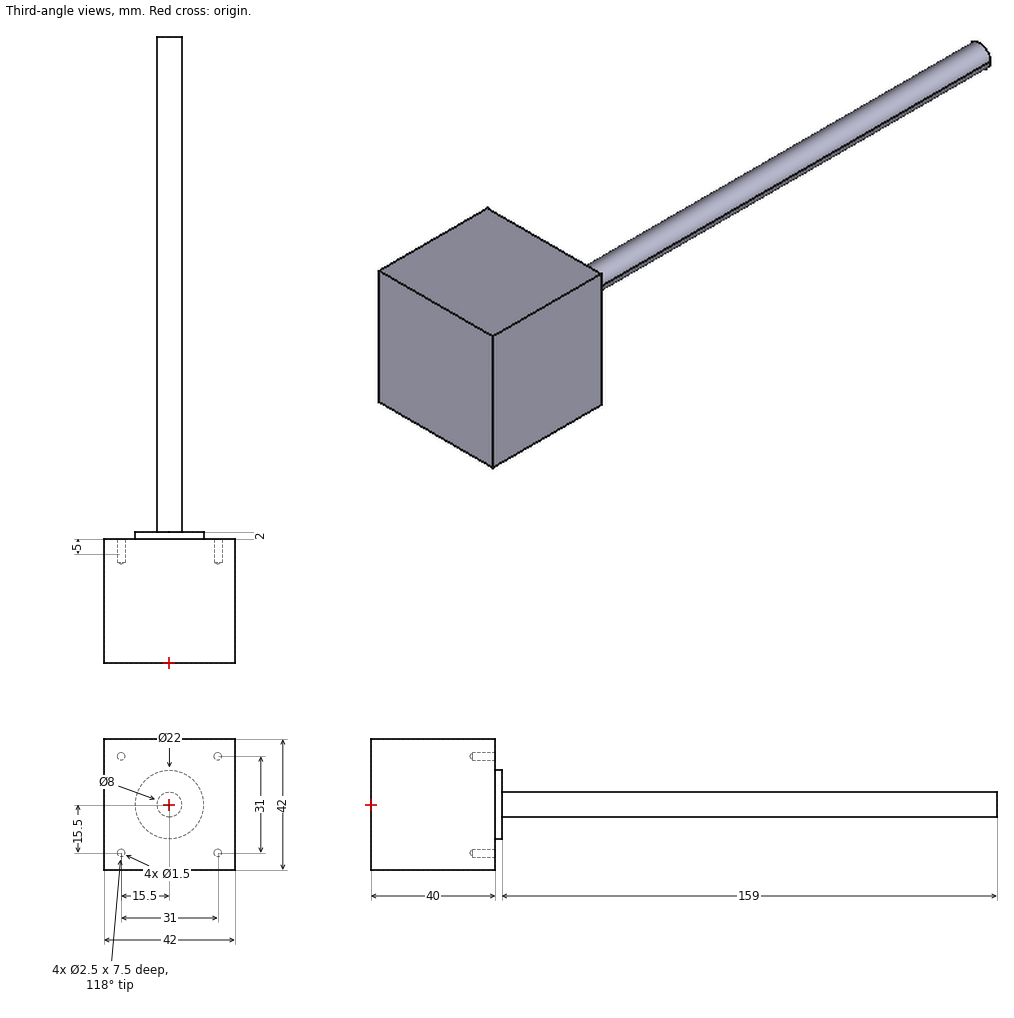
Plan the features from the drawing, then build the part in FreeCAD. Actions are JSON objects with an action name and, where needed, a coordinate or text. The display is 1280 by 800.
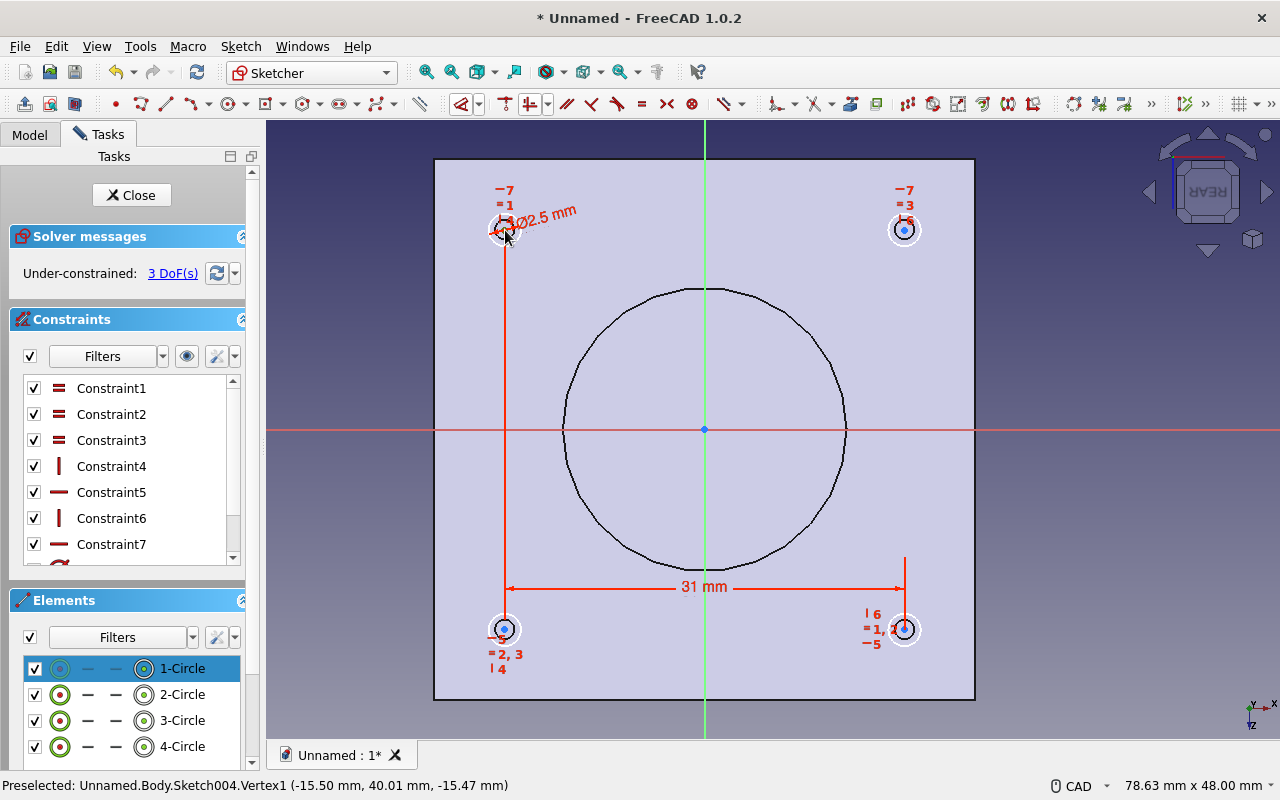
{"action": "left_click", "coordinate": [905, 630]}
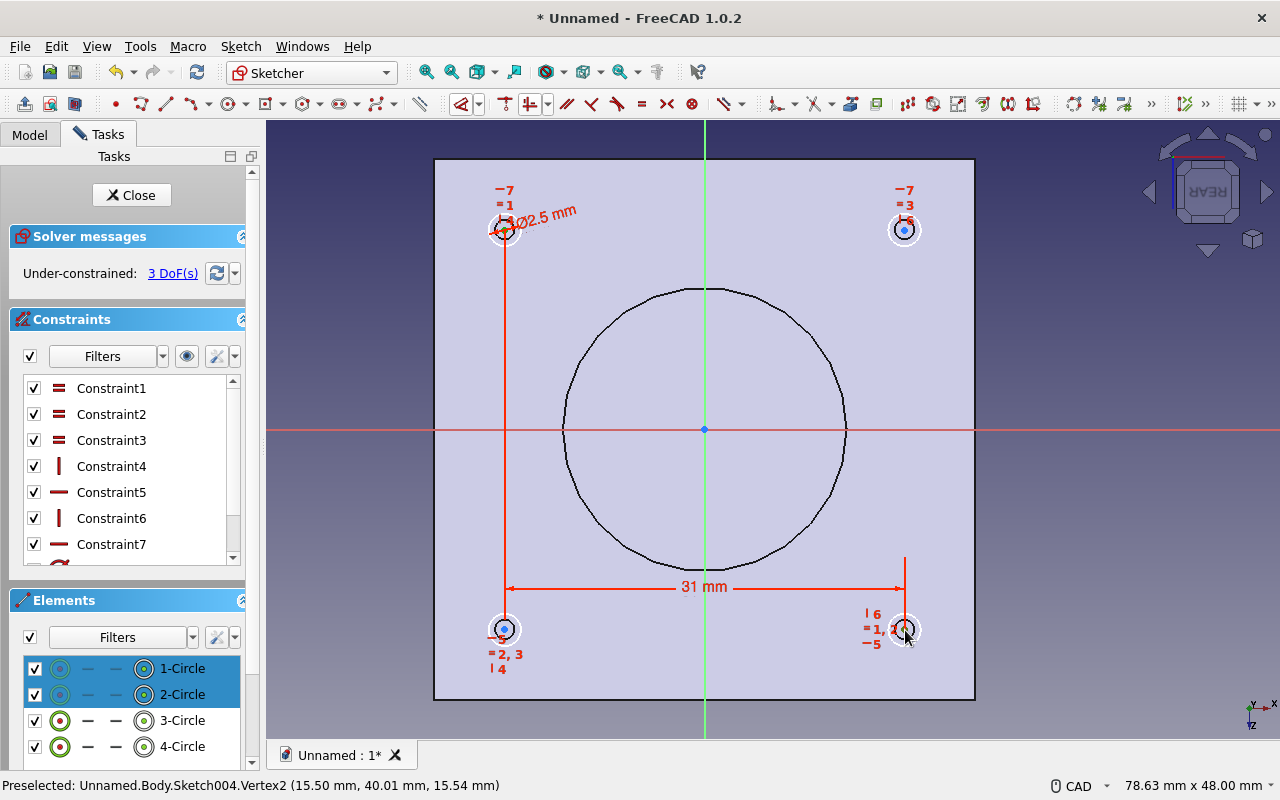
{"action": "key", "text": "i"}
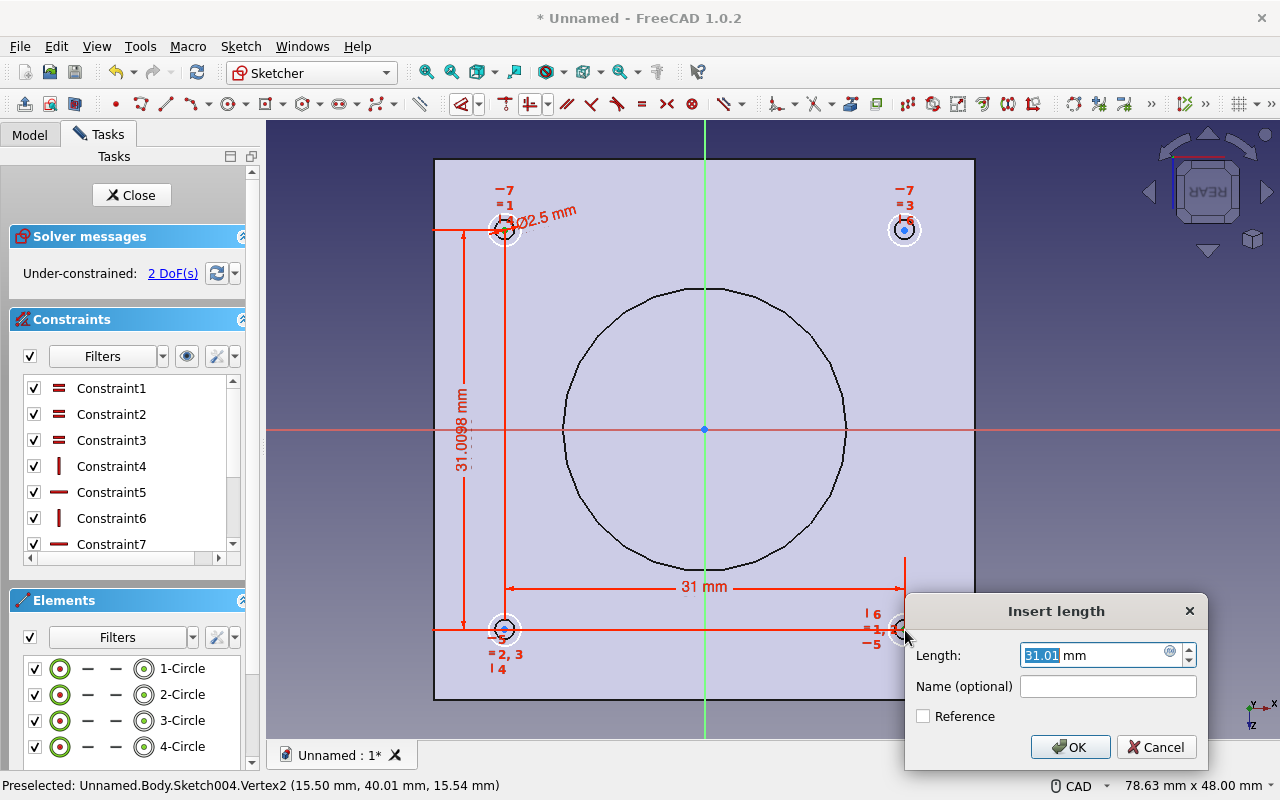
{"action": "type", "text": "31"}
{"action": "key", "text": "Return"}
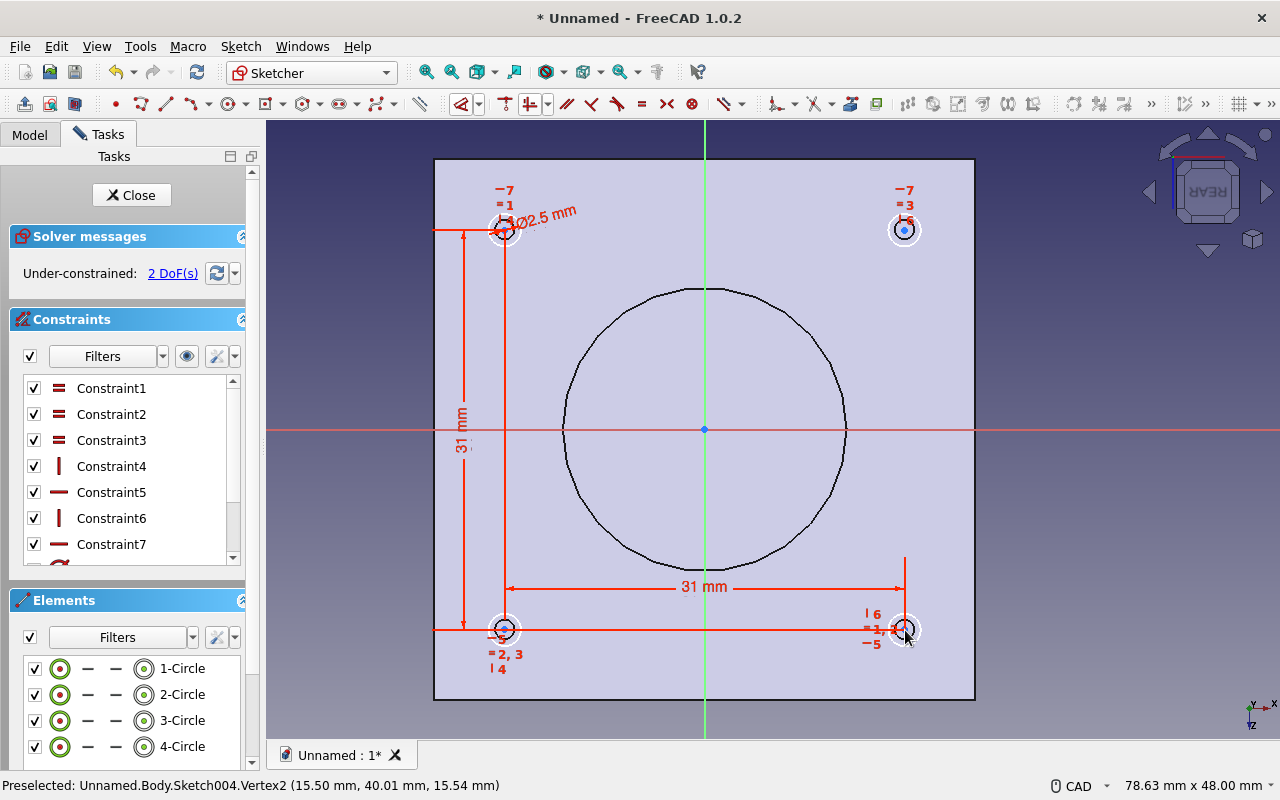
{"action": "left_click", "coordinate": [505, 230]}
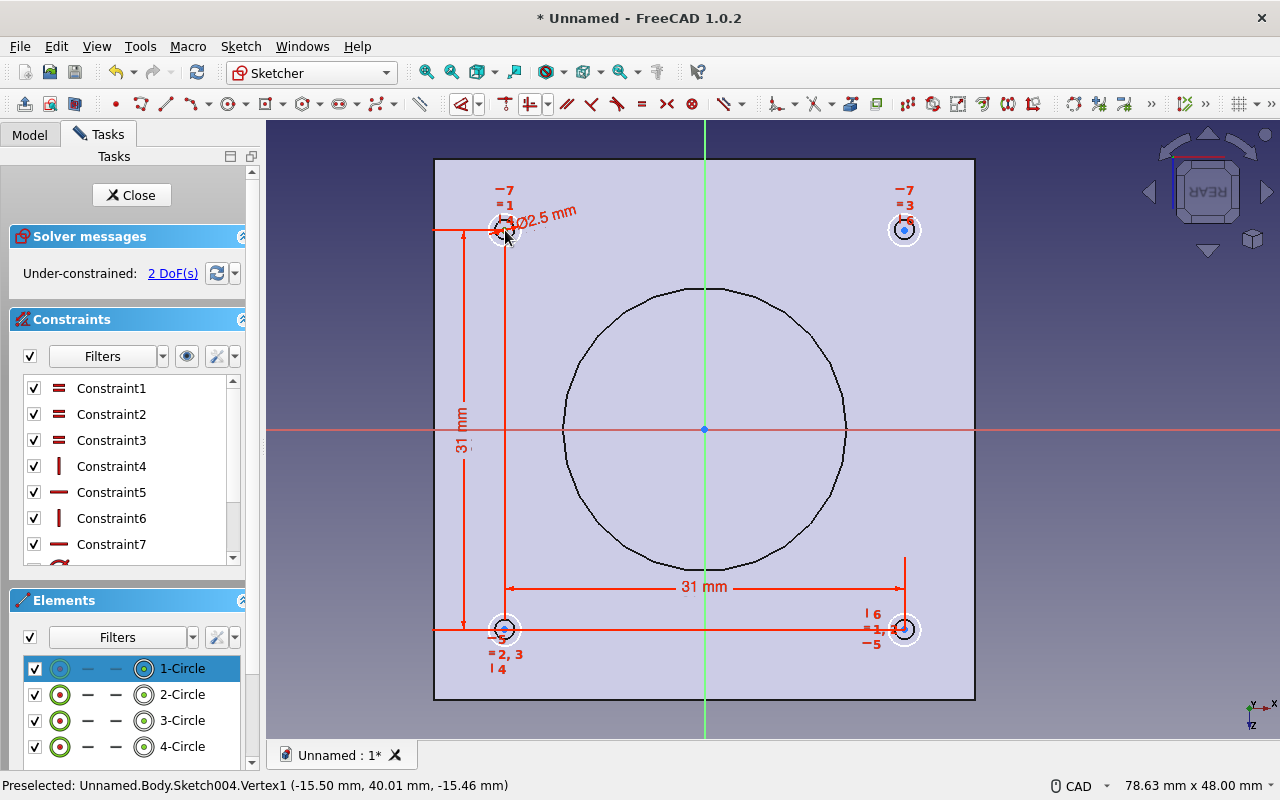
{"action": "key", "text": "l"}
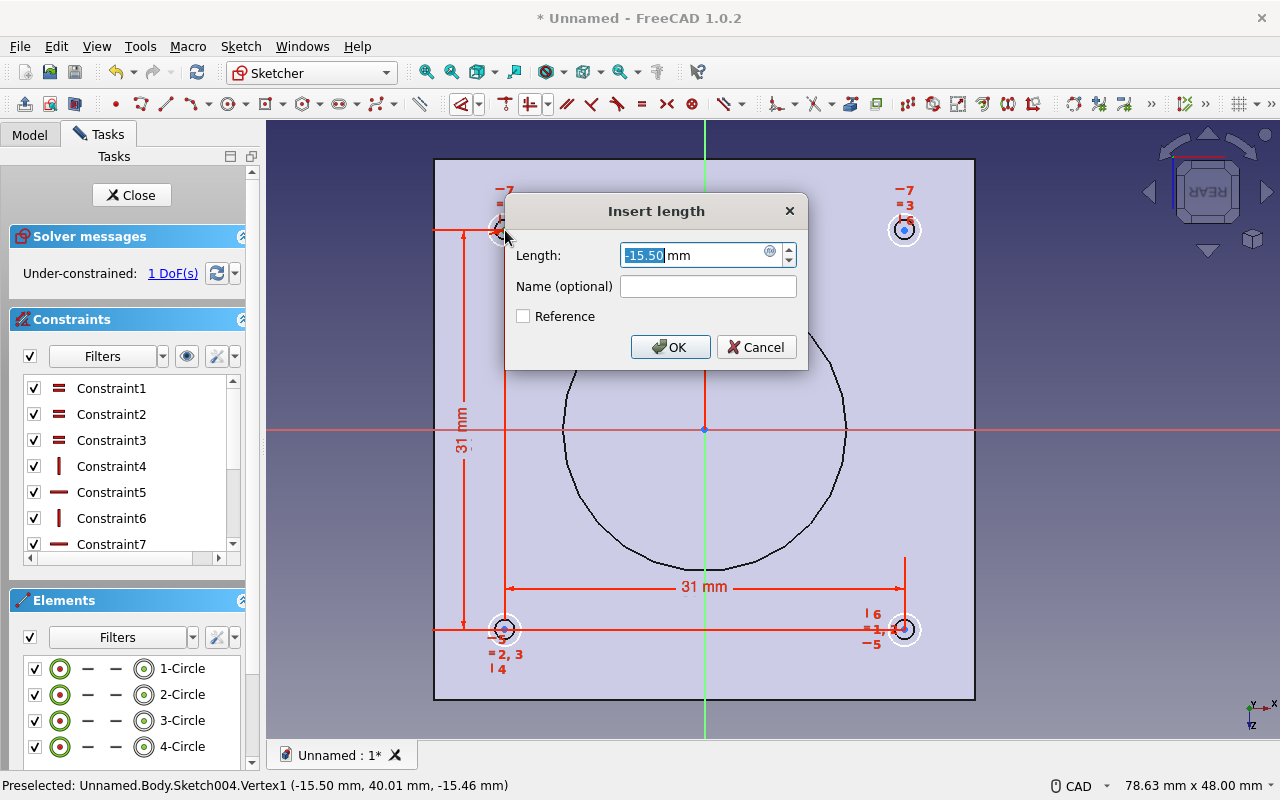
{"action": "type", "text": "-15.5"}
{"action": "key", "text": "Return"}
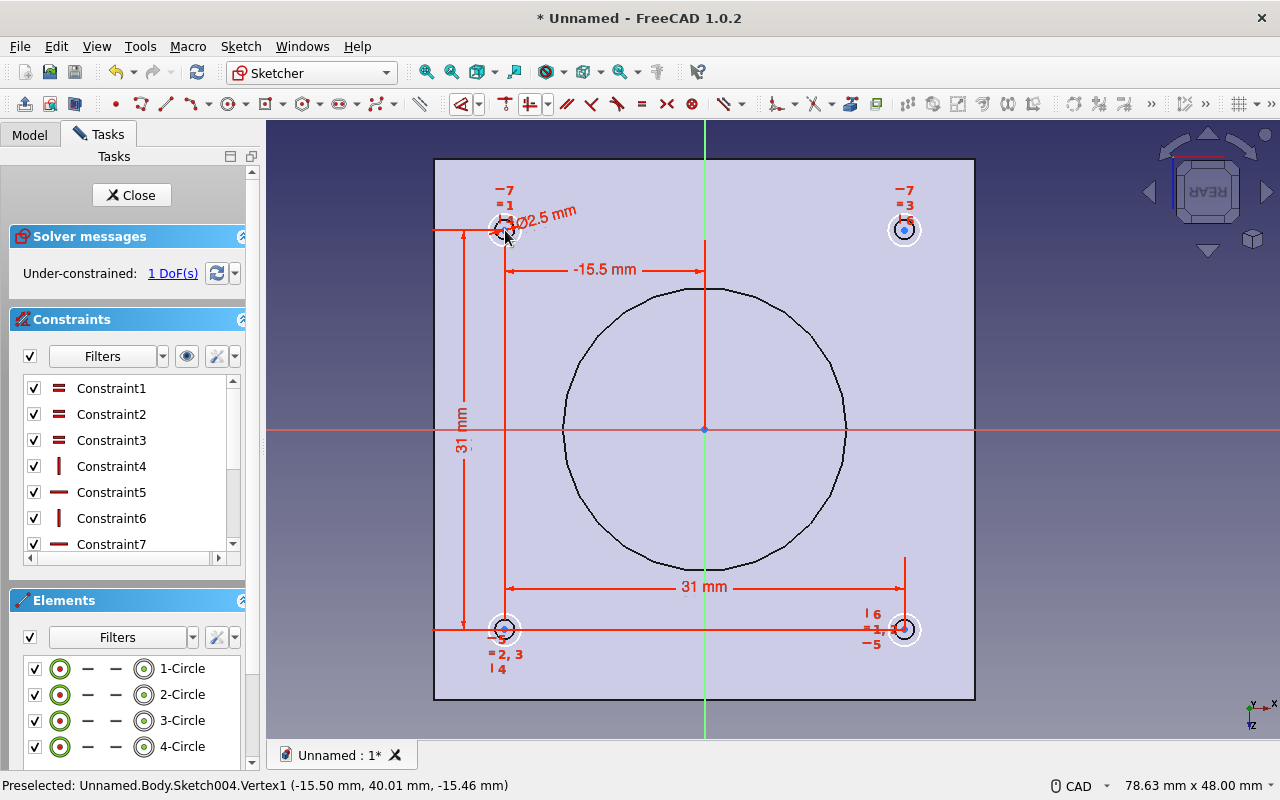
{"action": "left_click", "coordinate": [505, 230]}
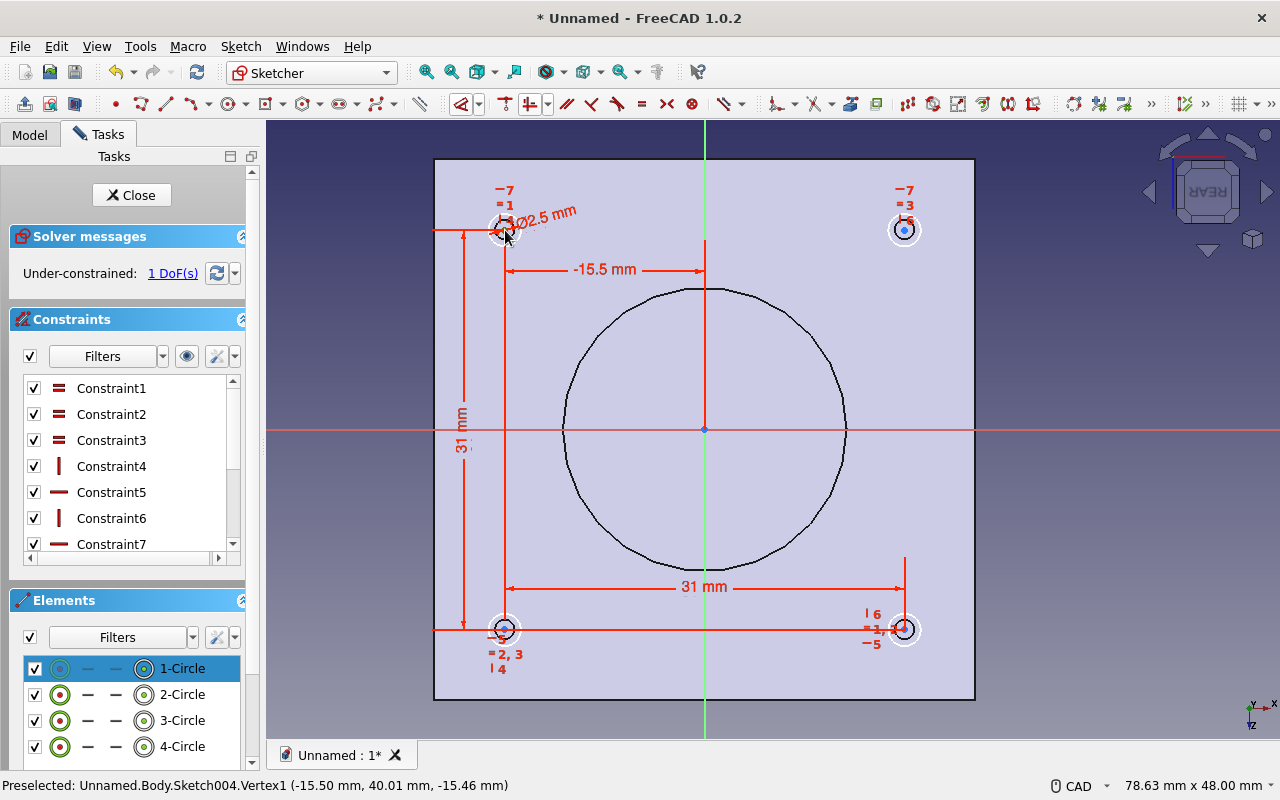
{"action": "key", "text": "i"}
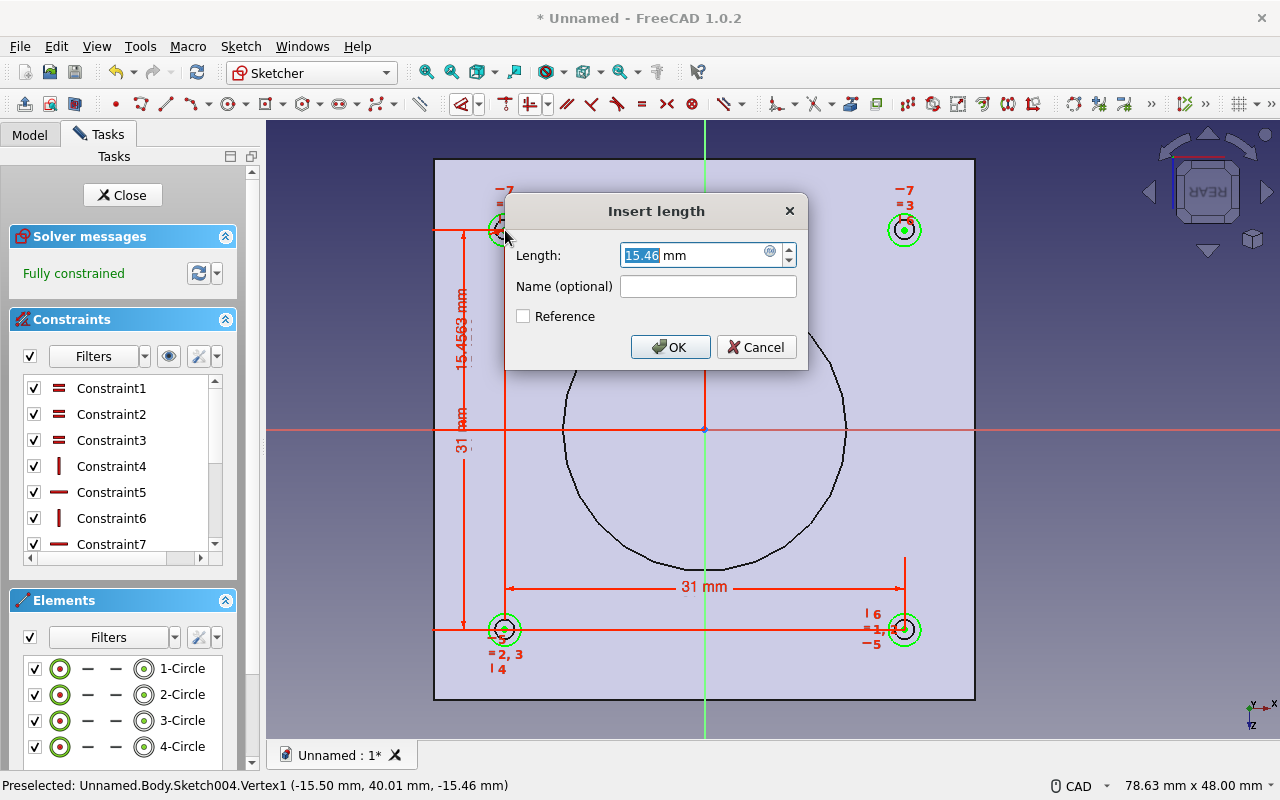
{"action": "type", "text": "15.5"}
{"action": "key", "text": "Return"}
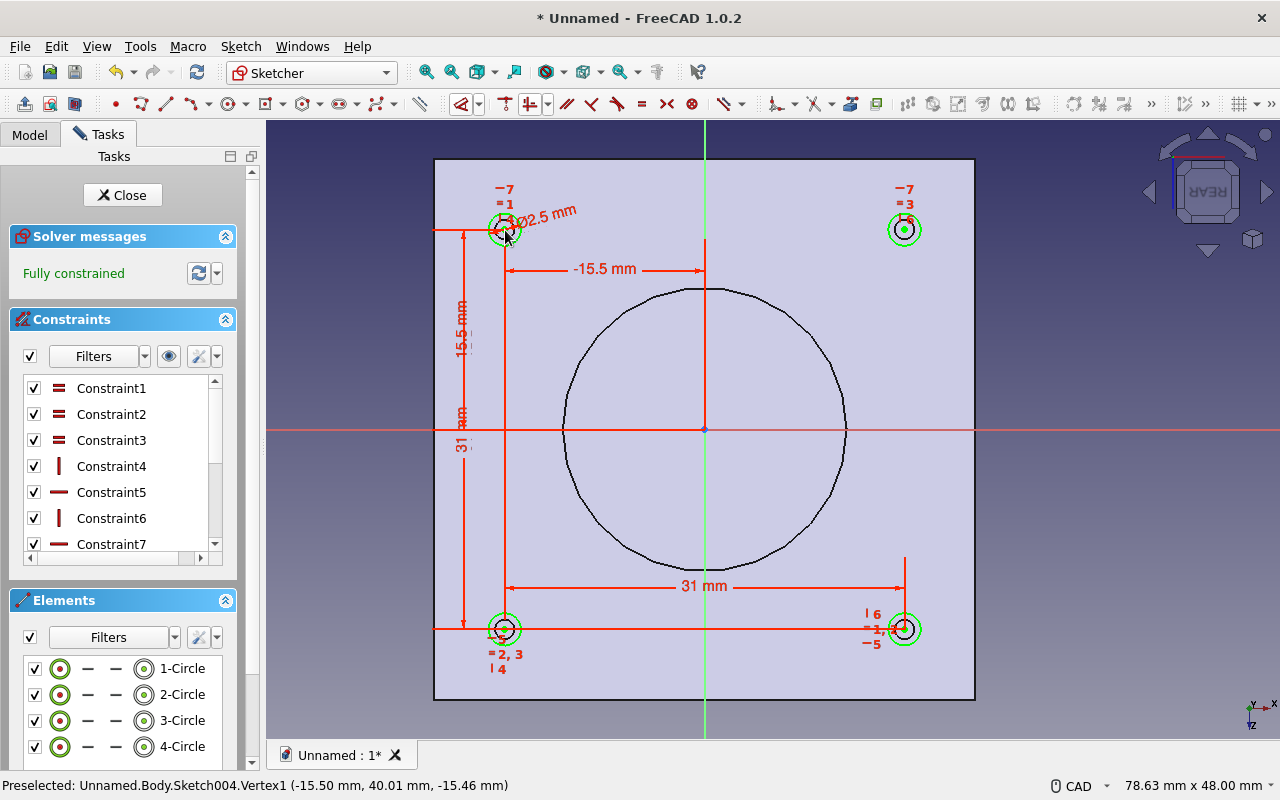
{"action": "left_click", "coordinate": [123, 195]}